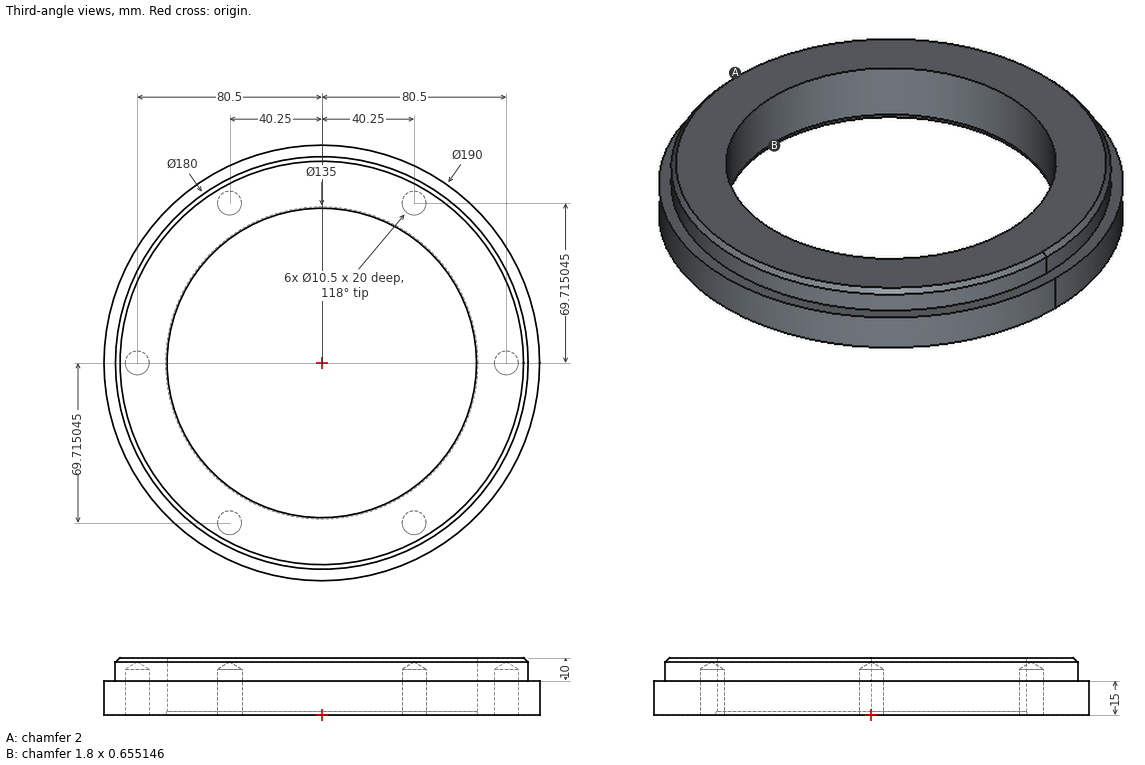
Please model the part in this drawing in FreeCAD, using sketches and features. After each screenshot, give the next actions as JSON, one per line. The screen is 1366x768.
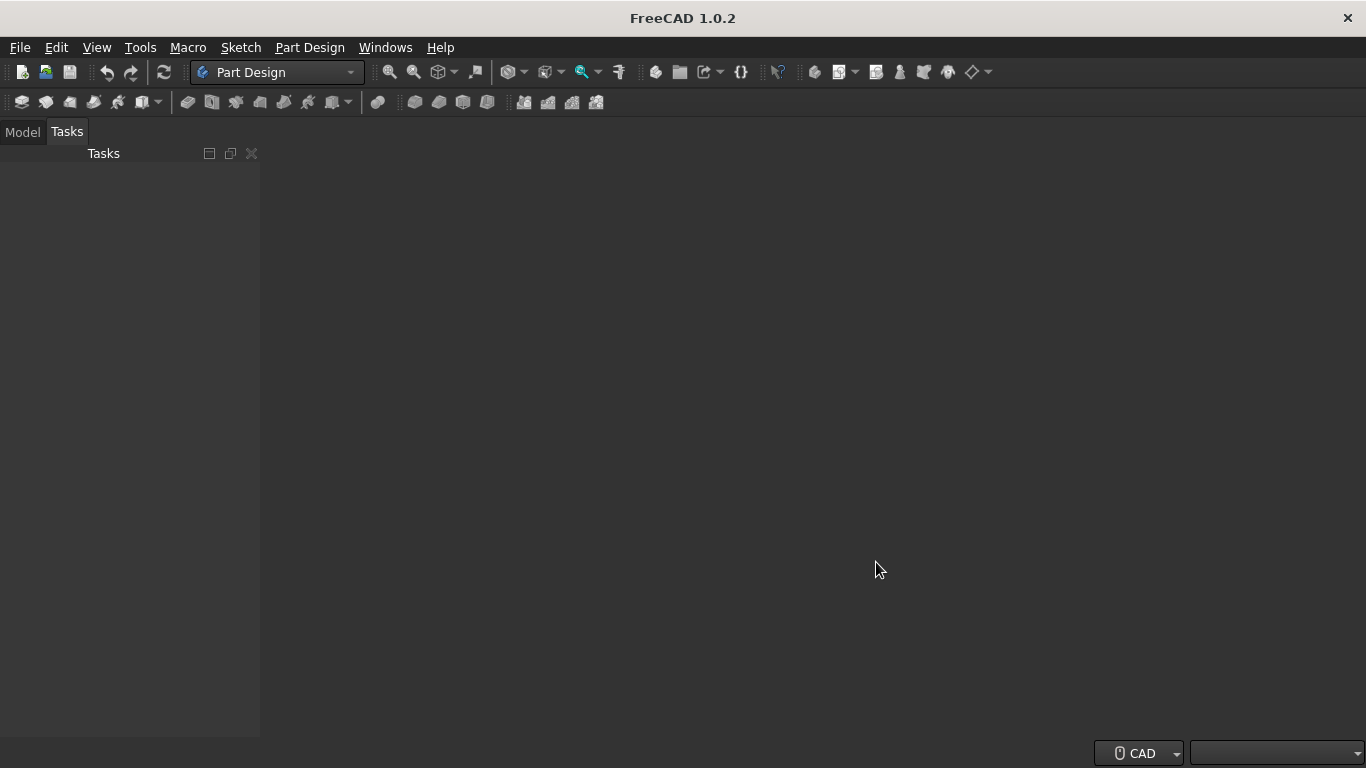
{"action": "left_click", "coordinate": [22, 72]}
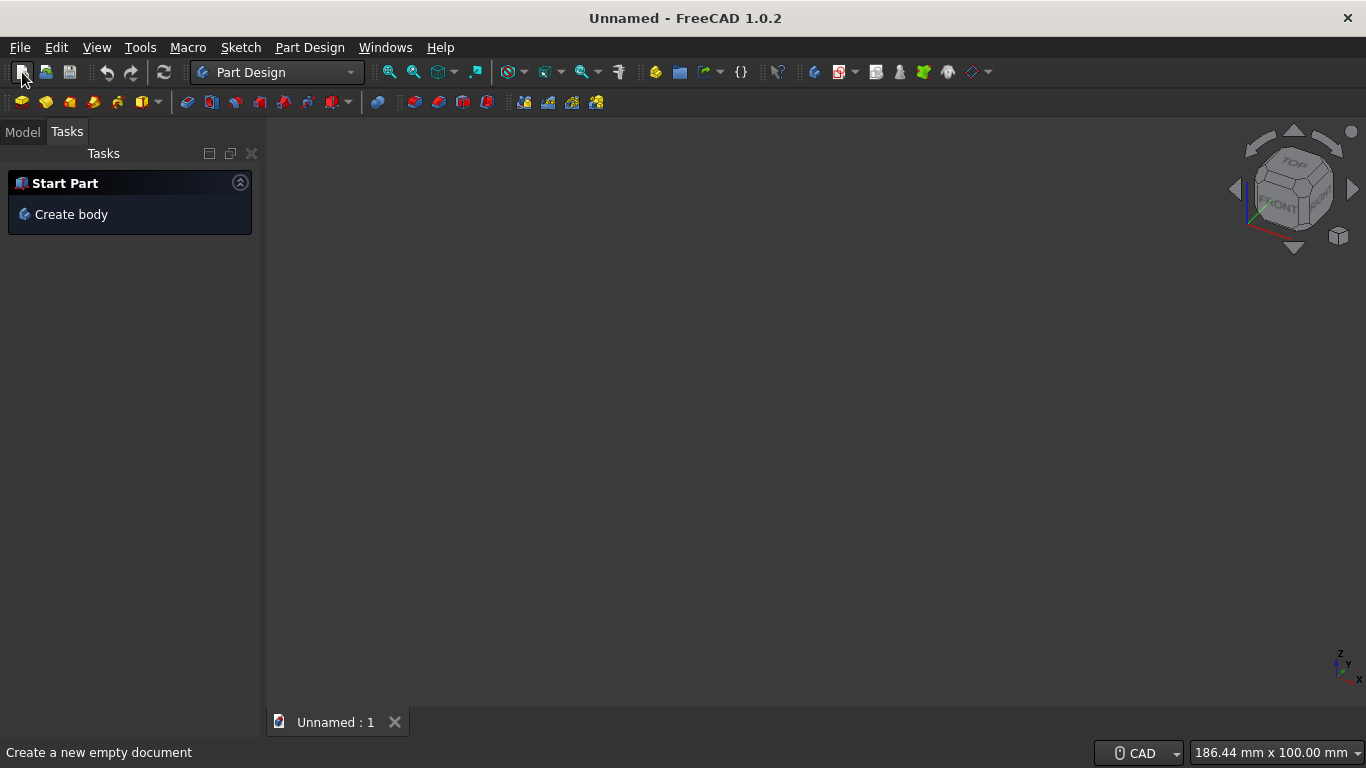
{"action": "left_click", "coordinate": [840, 72]}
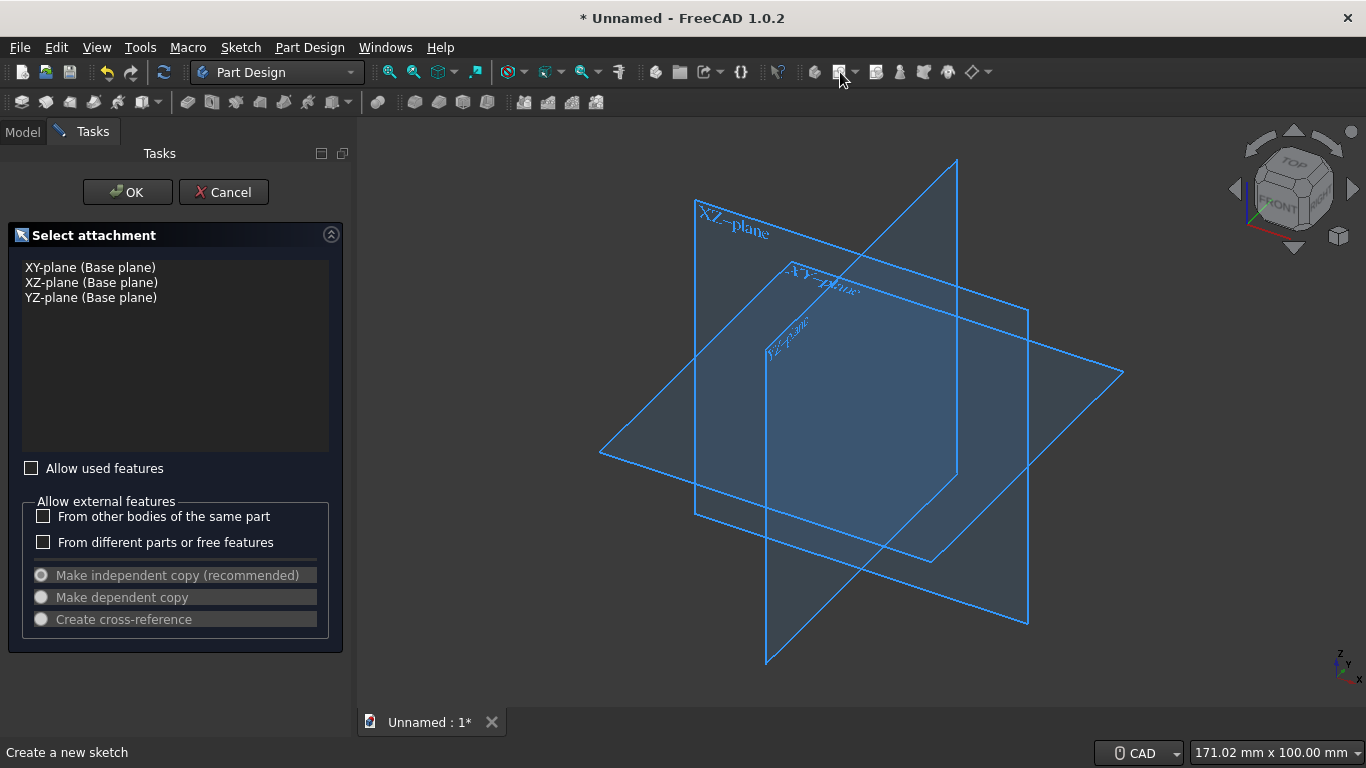
{"action": "left_click", "coordinate": [82, 268]}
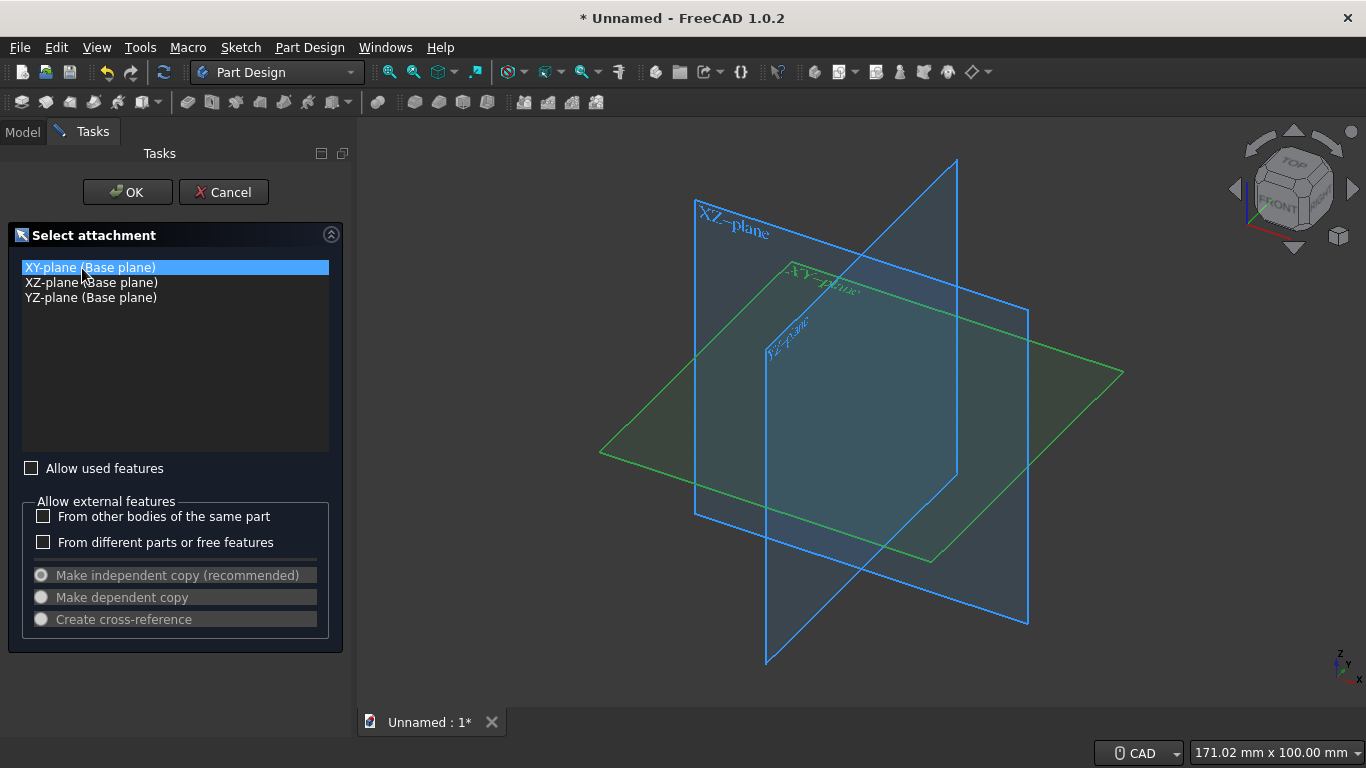
{"action": "left_click", "coordinate": [128, 192]}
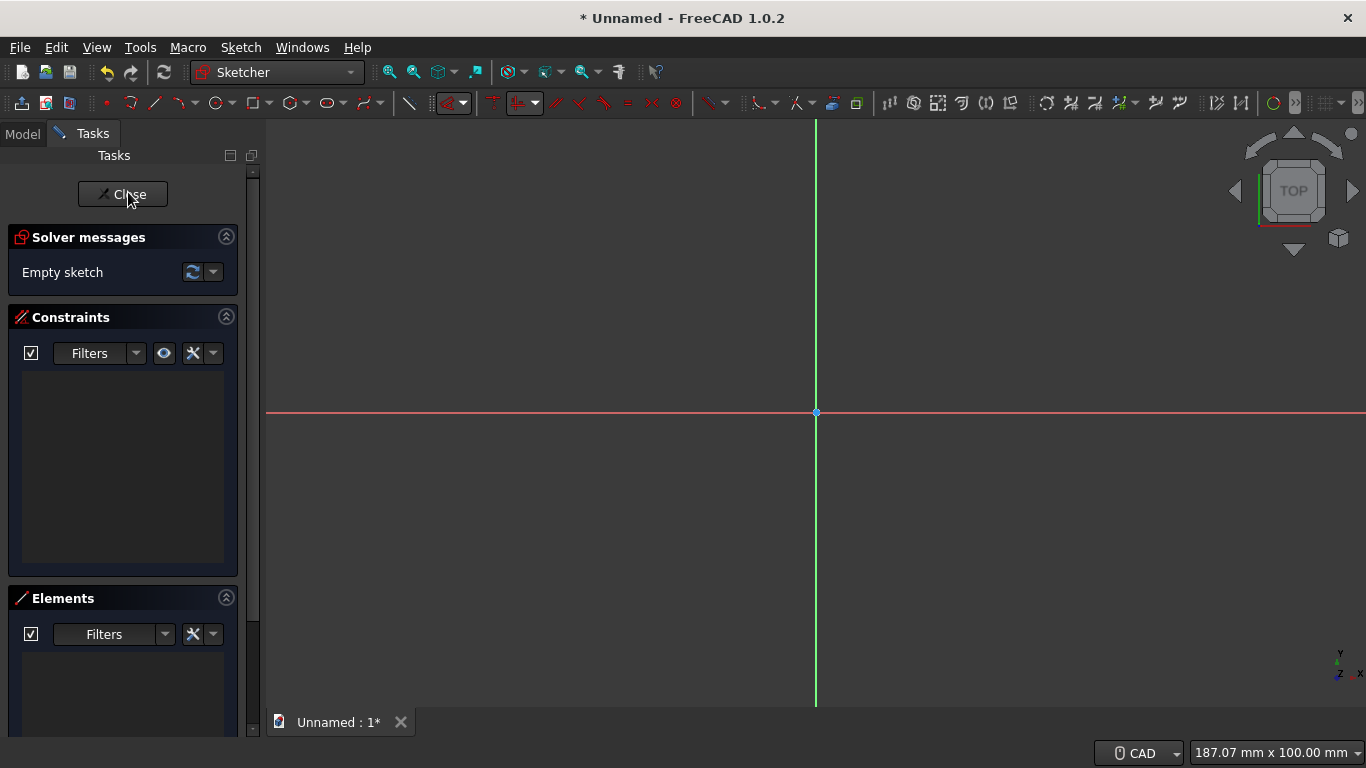
{"action": "scroll", "coordinate": [708, 413], "scroll_direction": "down", "scroll_amount": 5}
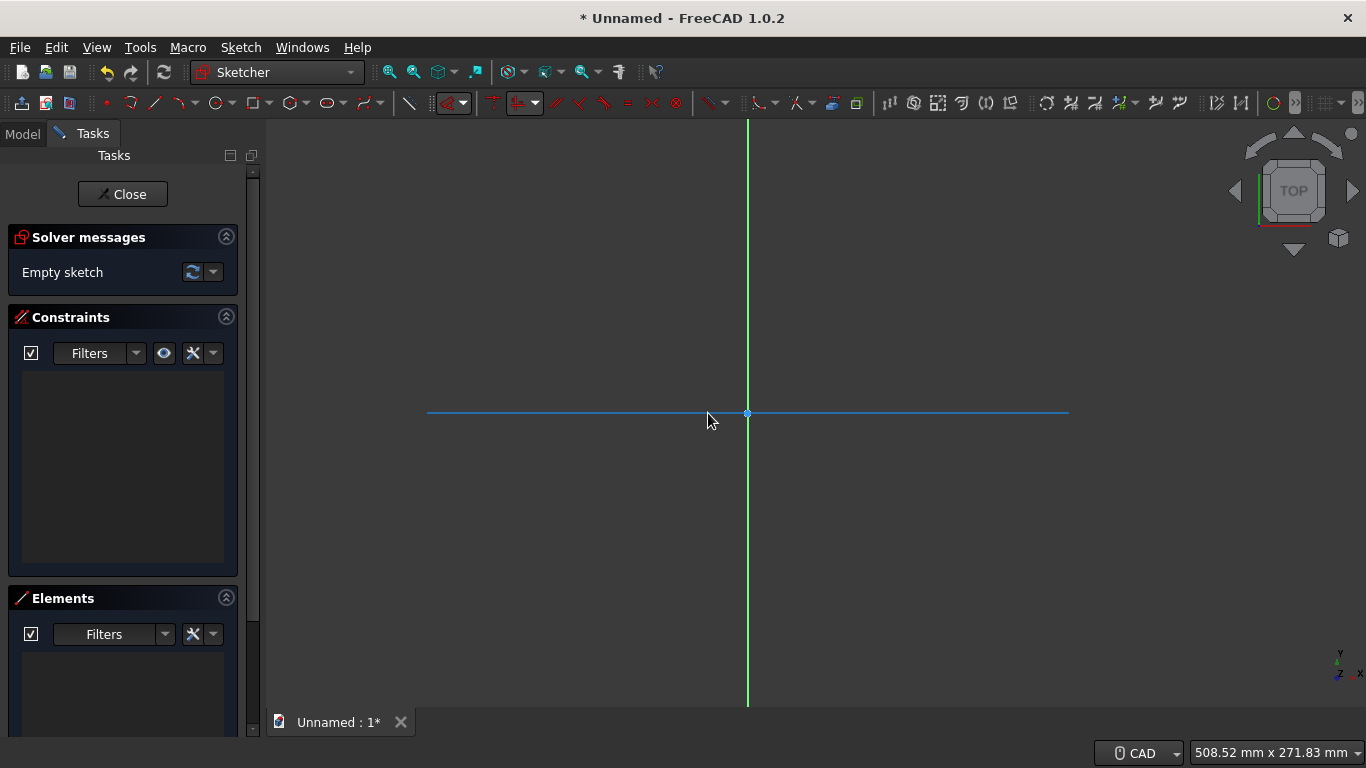
{"action": "left_click", "coordinate": [216, 104]}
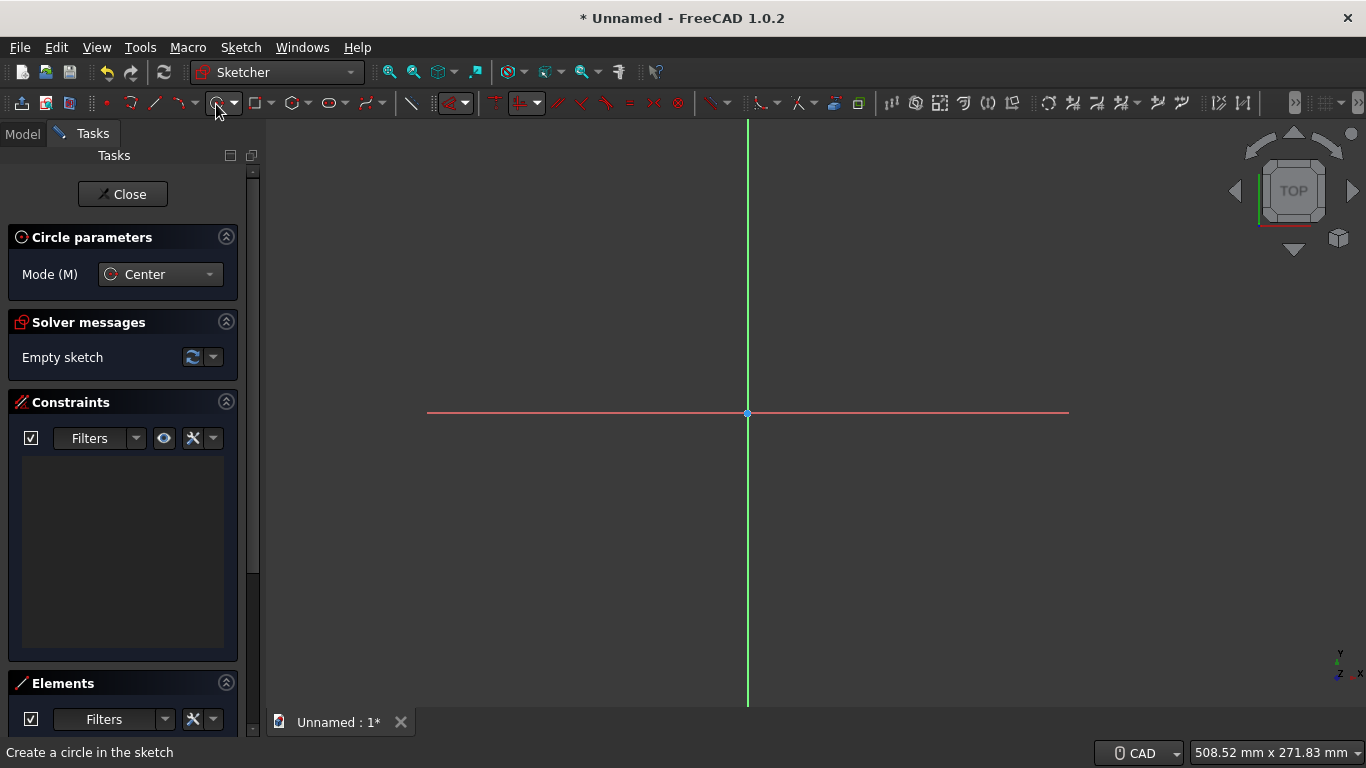
{"action": "left_click", "coordinate": [748, 413]}
{"action": "left_click", "coordinate": [893, 268]}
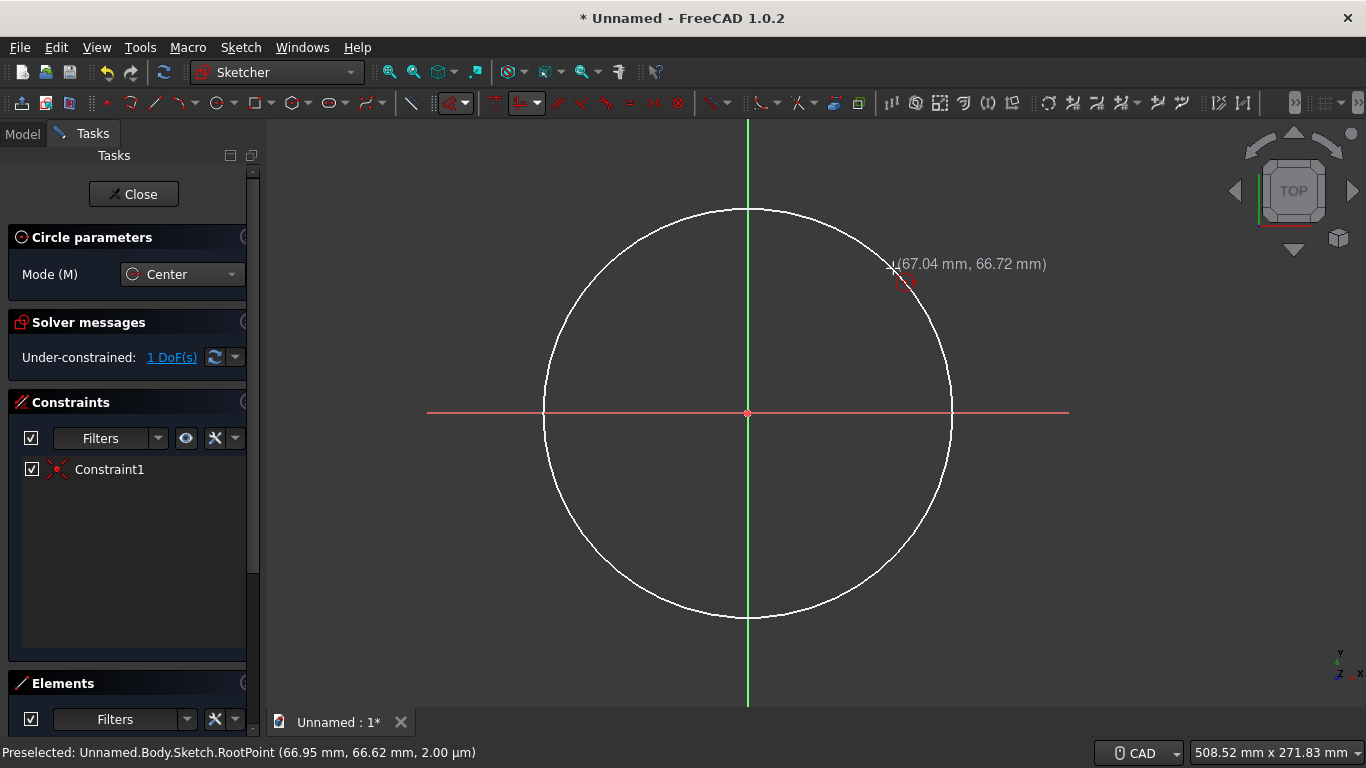
{"action": "left_click", "coordinate": [748, 413]}
{"action": "left_click", "coordinate": [851, 310]}
{"action": "key", "text": "Escape"}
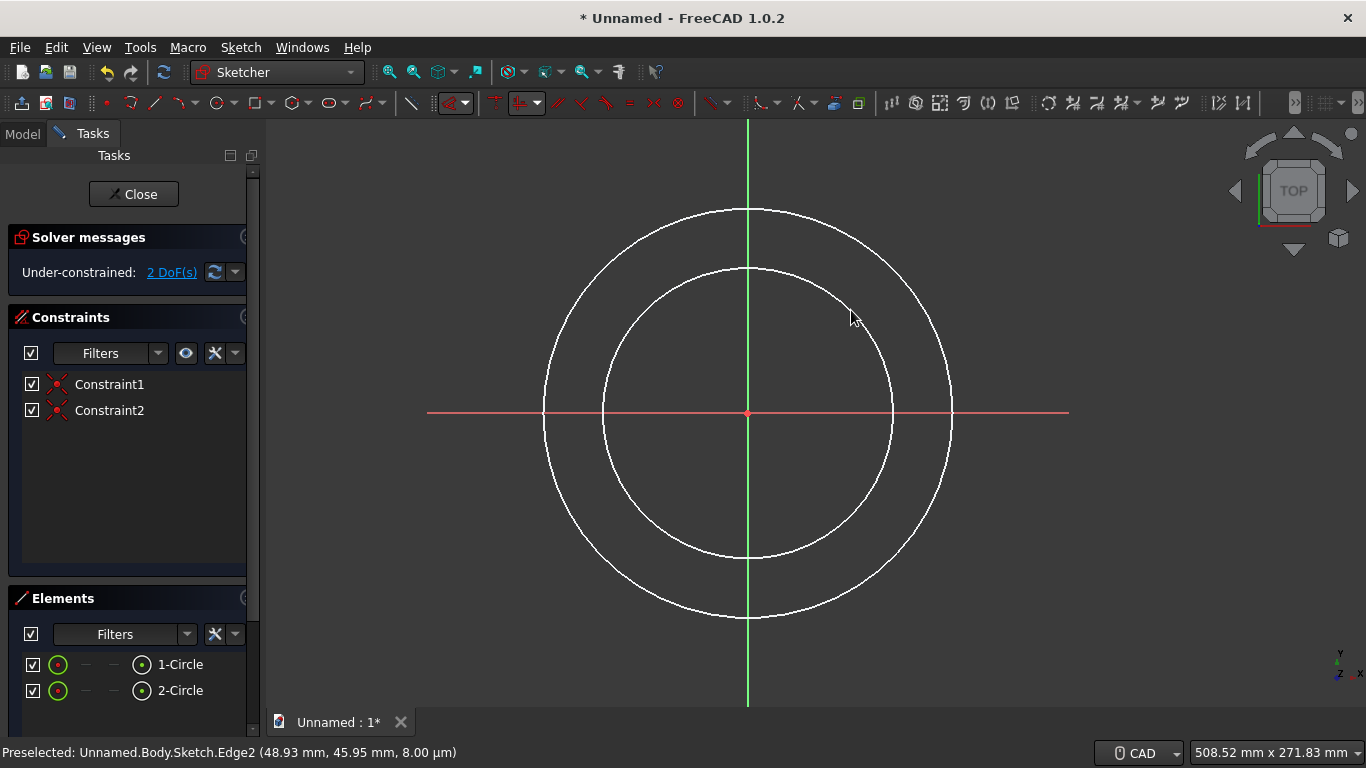
{"action": "left_click", "coordinate": [450, 104]}